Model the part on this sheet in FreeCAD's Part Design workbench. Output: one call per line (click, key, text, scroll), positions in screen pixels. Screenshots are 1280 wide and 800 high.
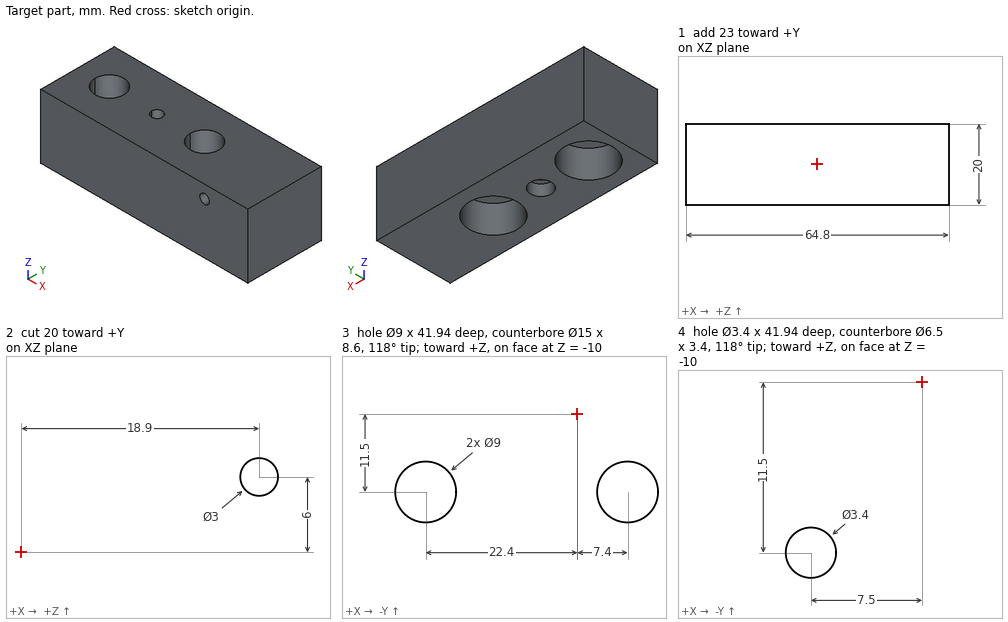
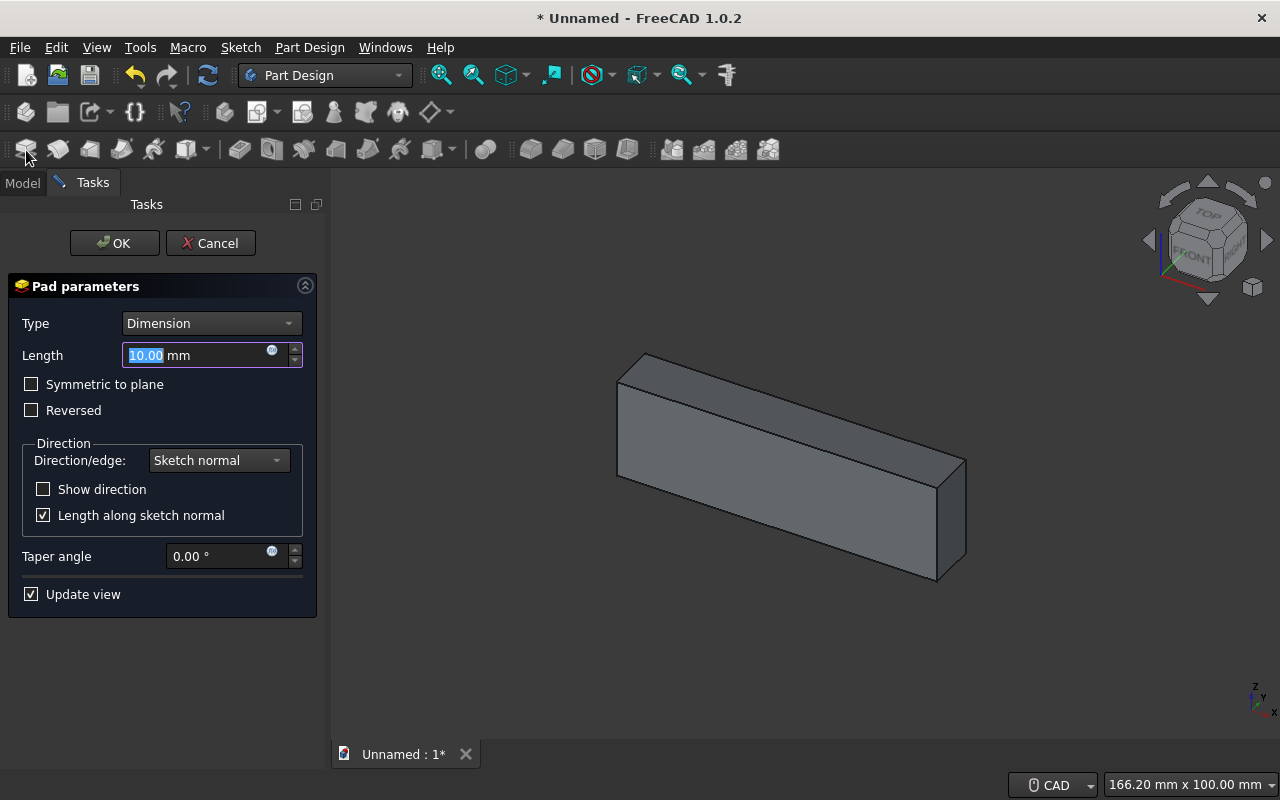
text(23)
key(Tab)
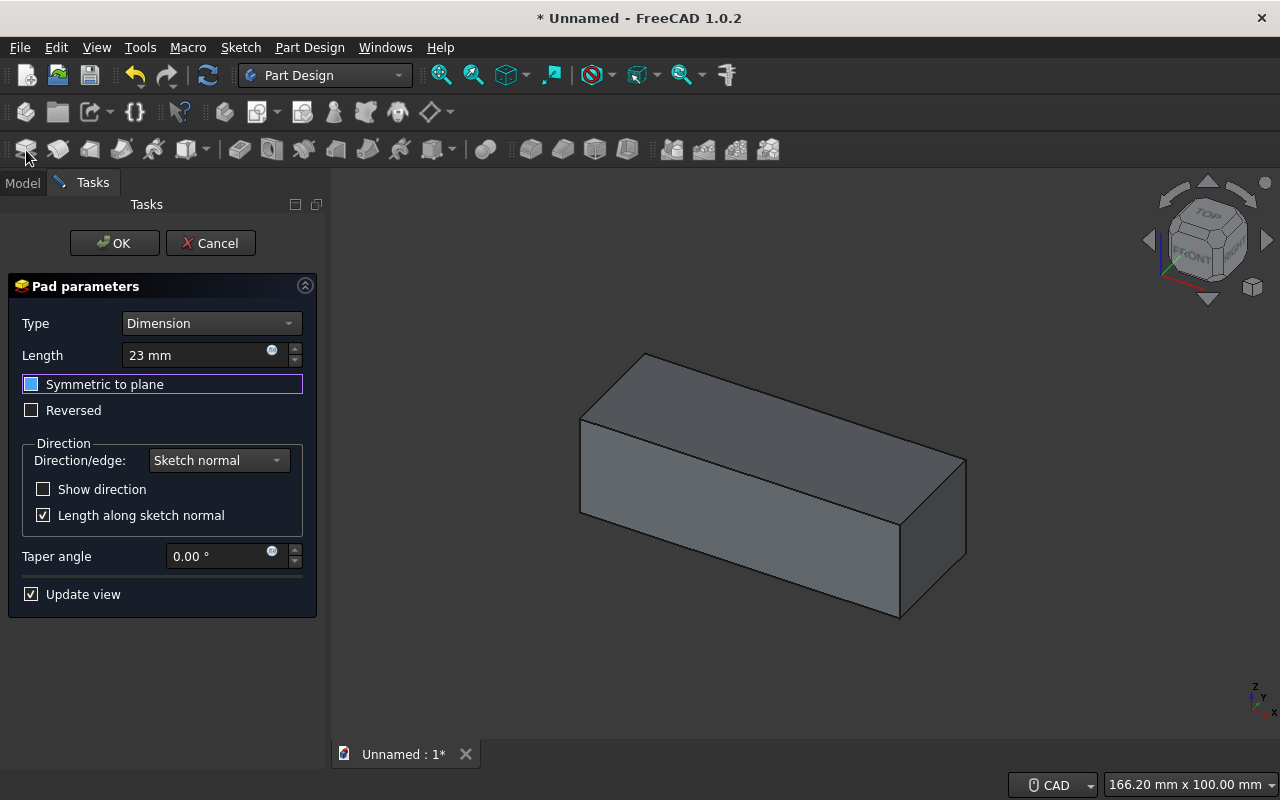
click(30, 410)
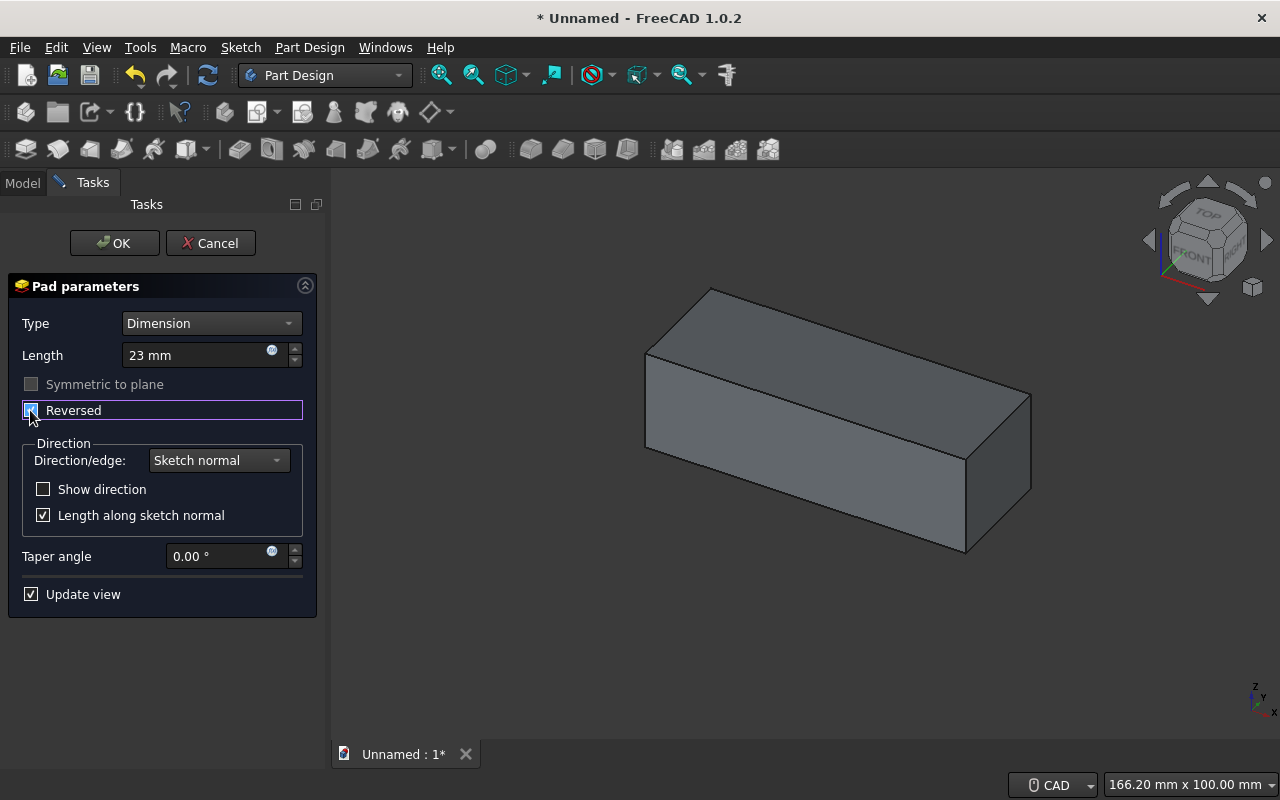
click(115, 243)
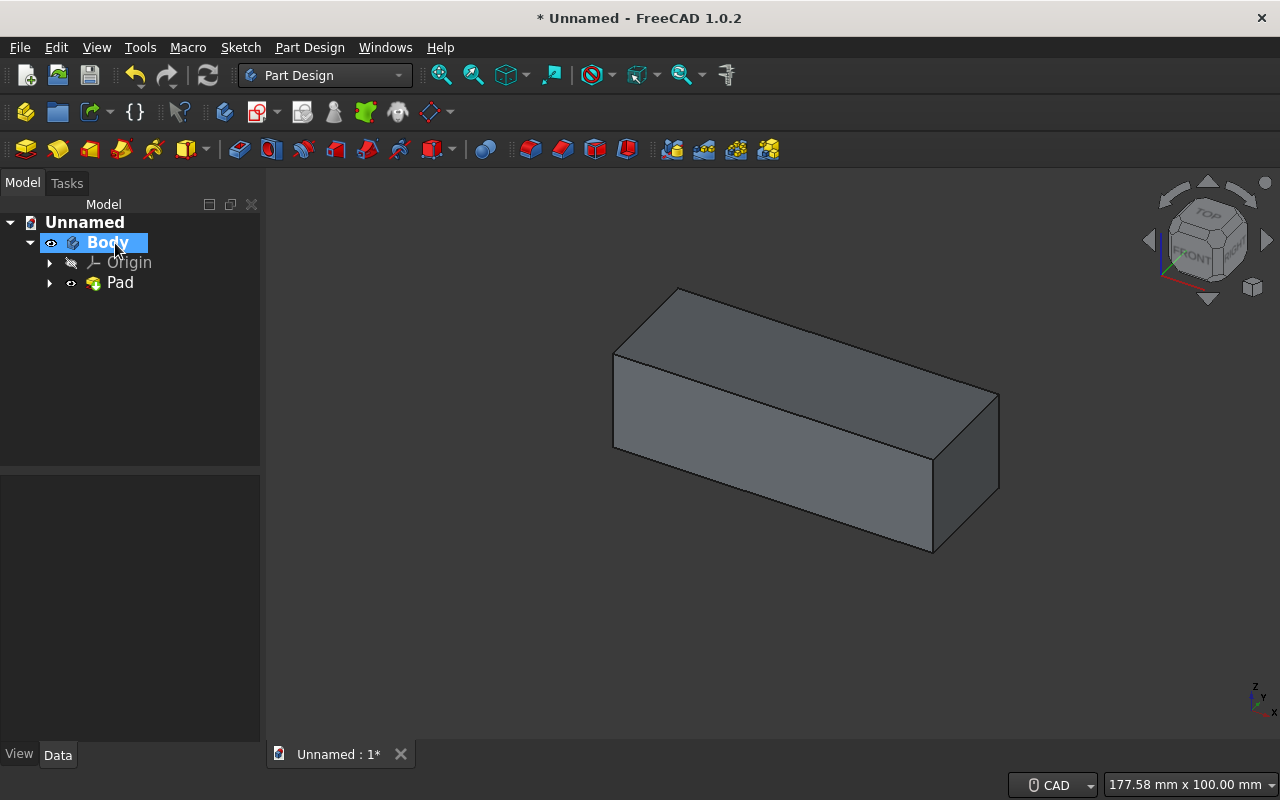
click(258, 112)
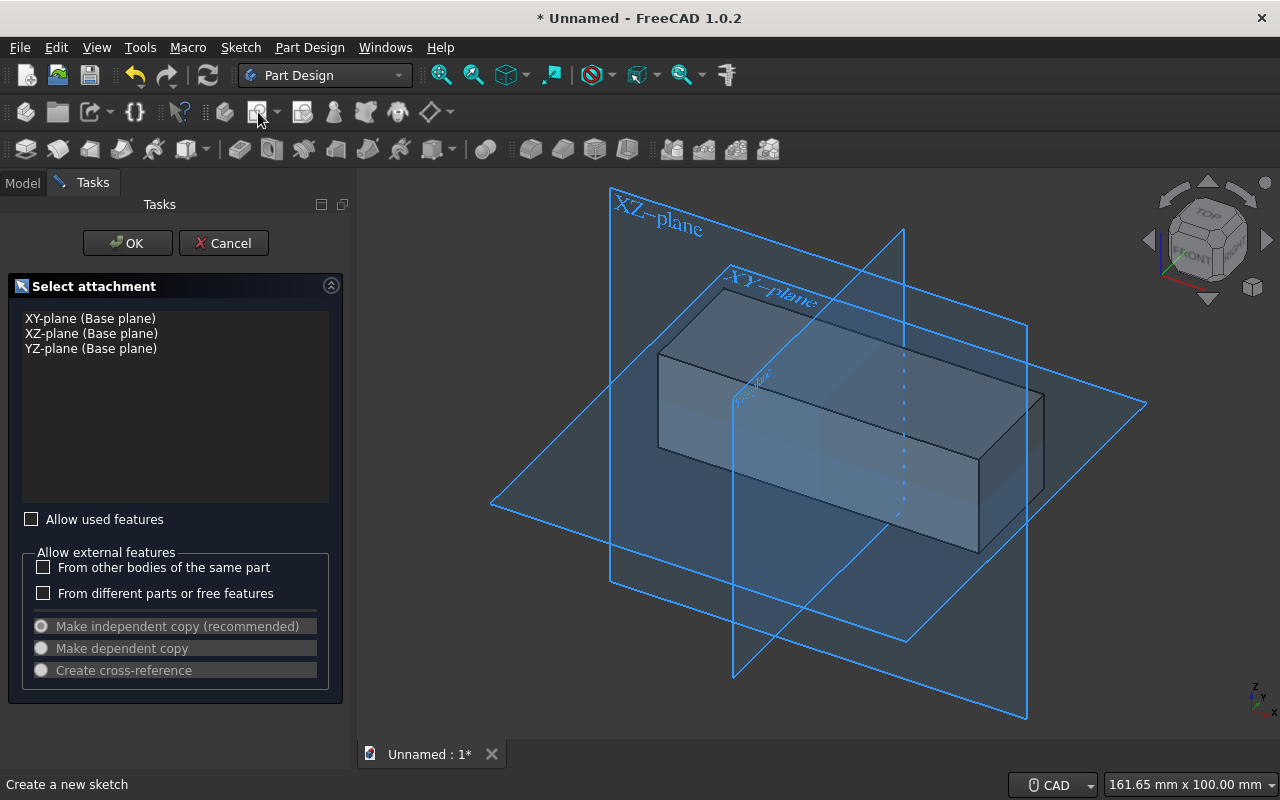
click(82, 334)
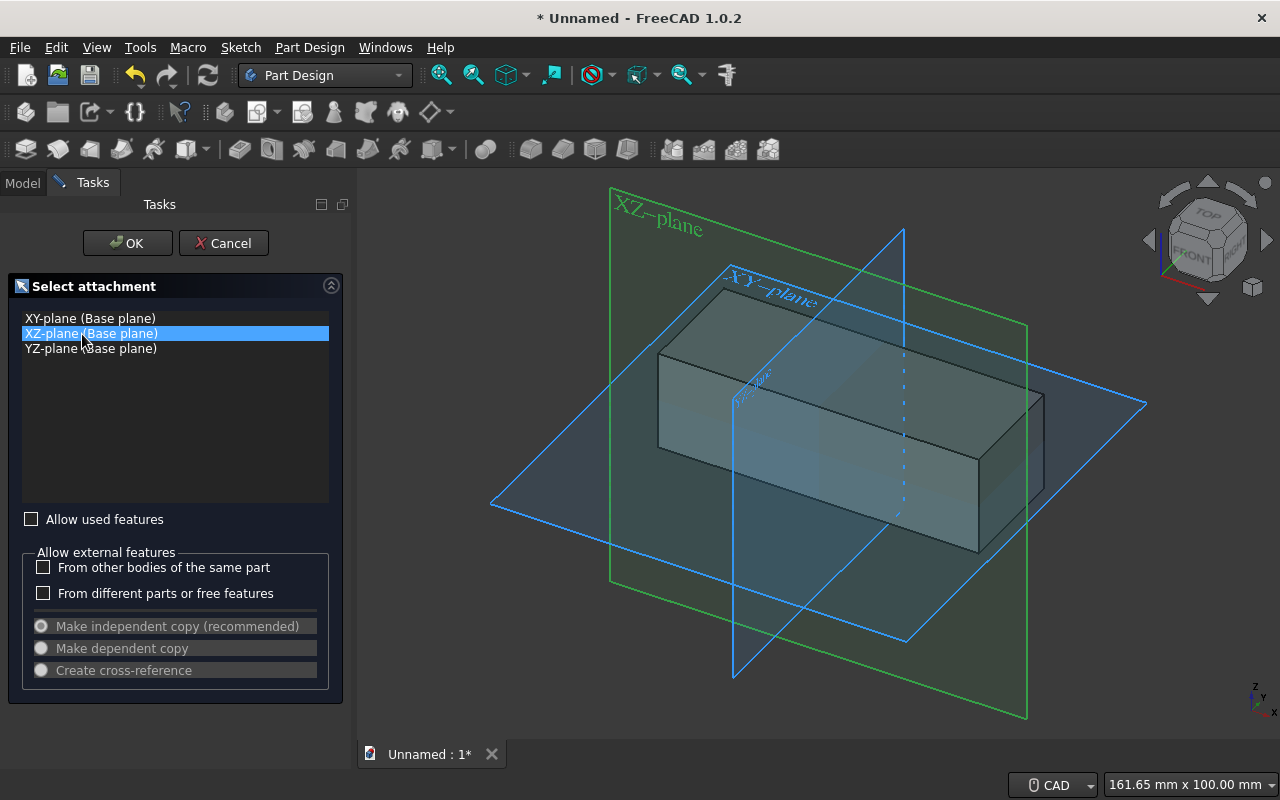
click(128, 243)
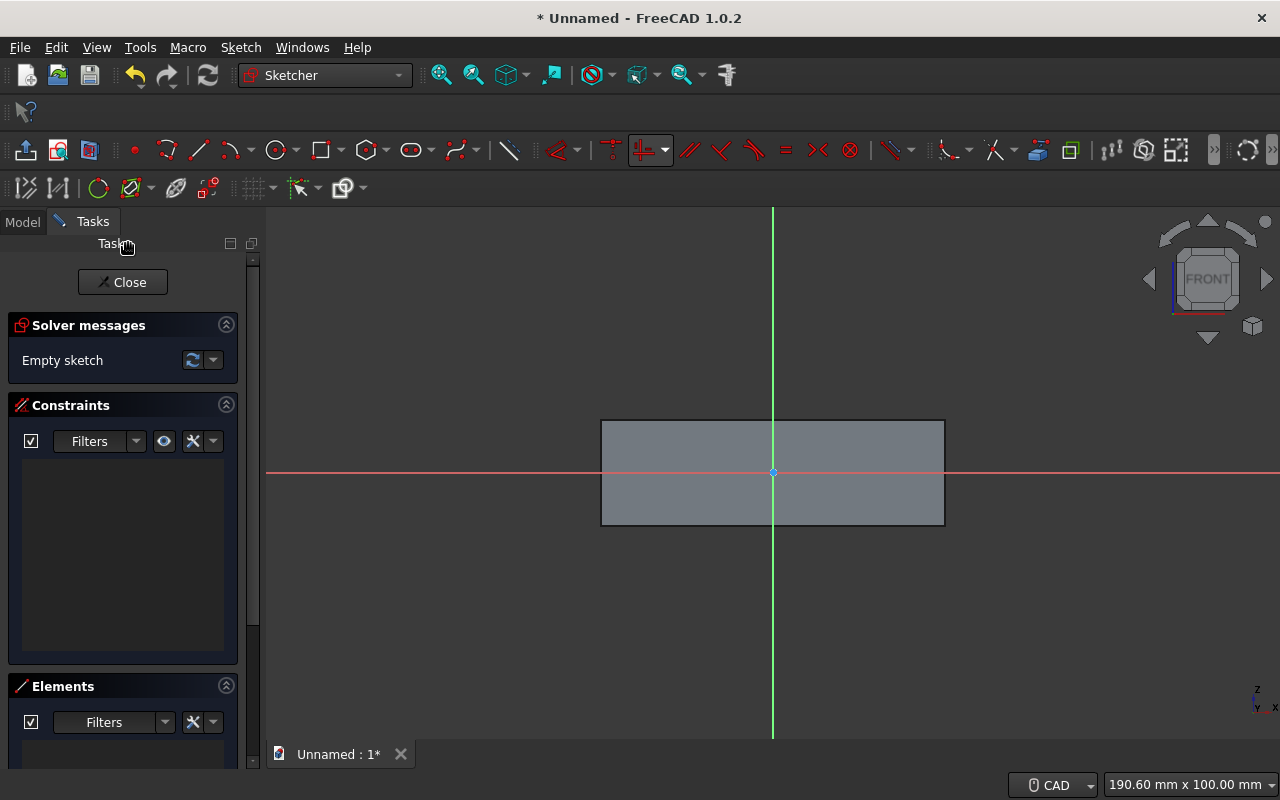
scroll(882, 439, up, 15)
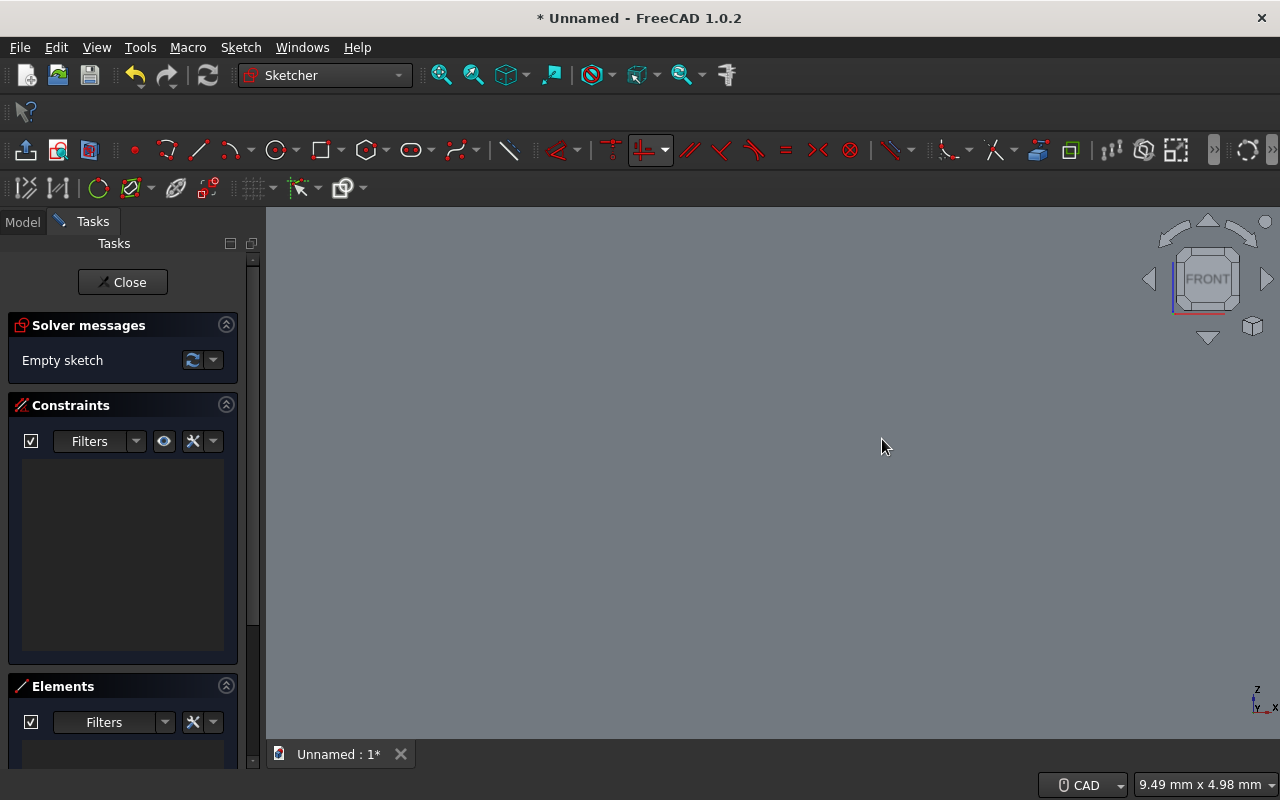
click(276, 150)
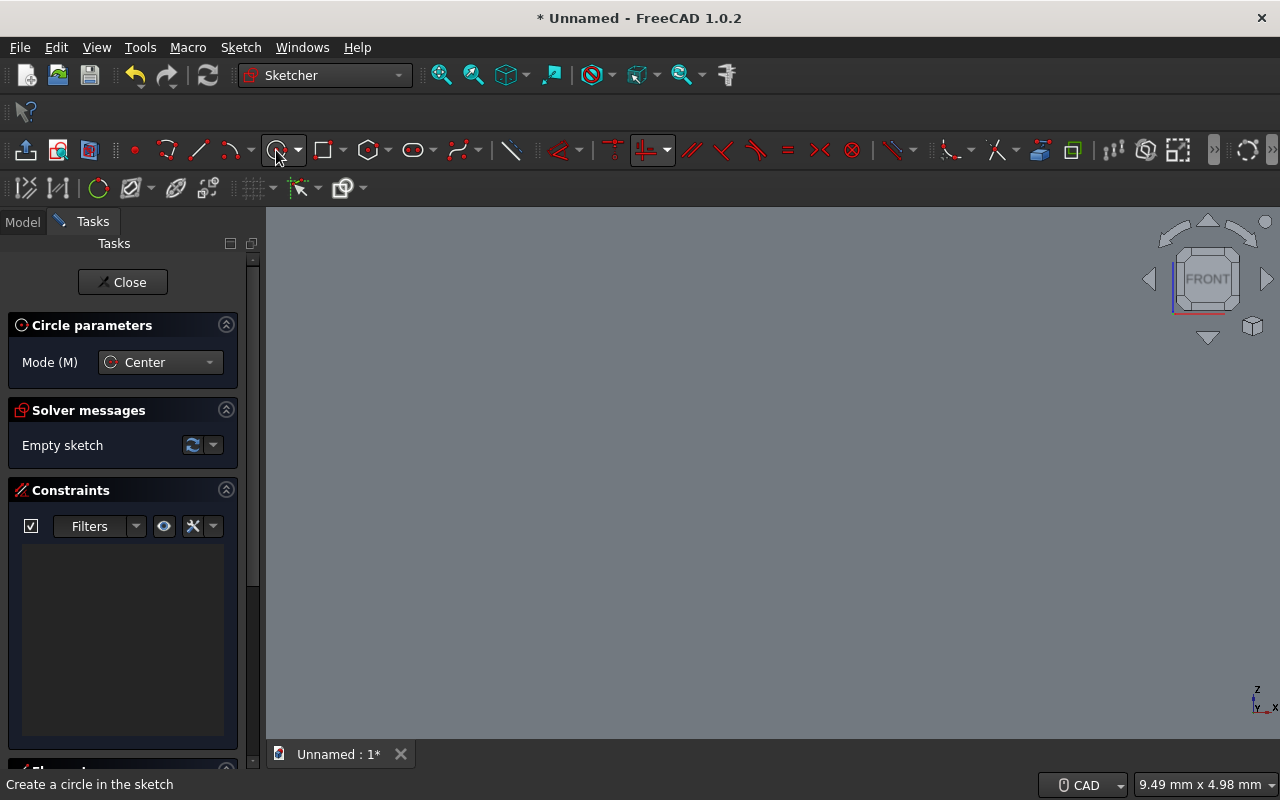
click(701, 472)
move(814, 359)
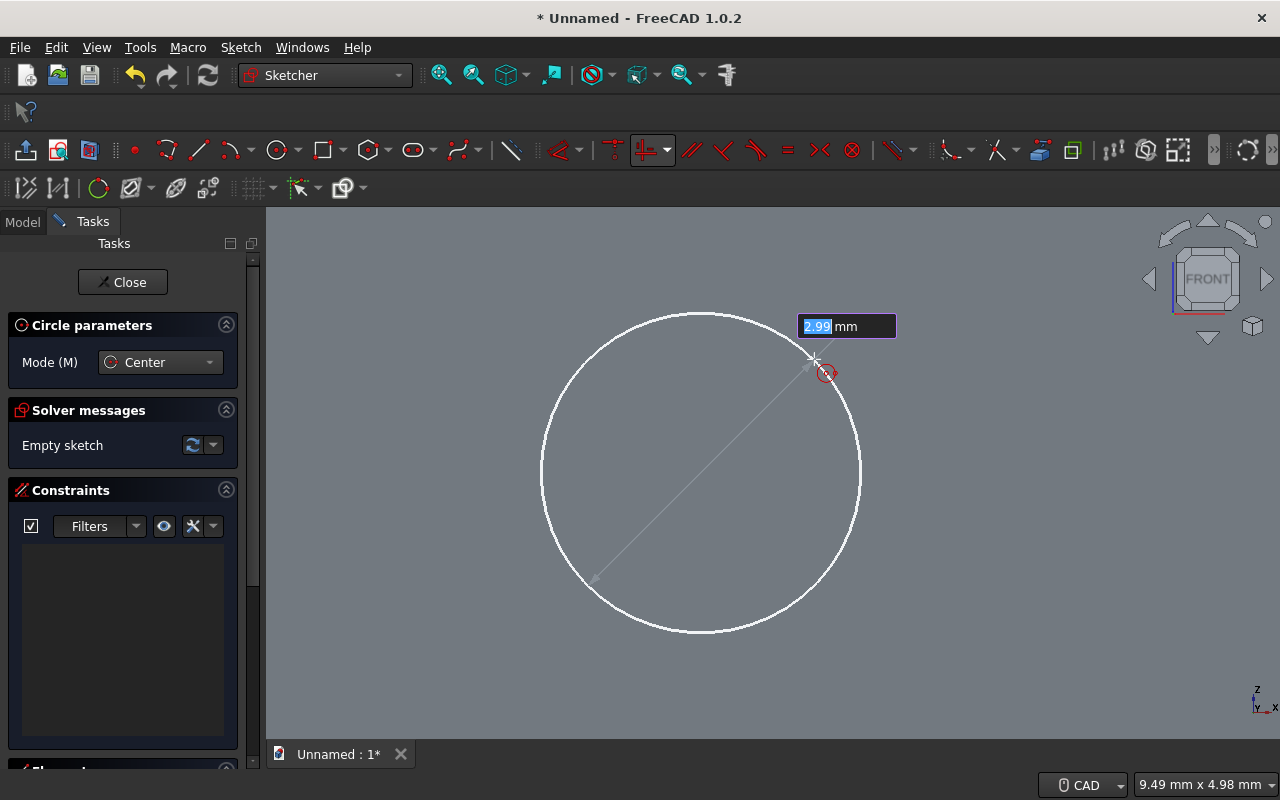
text(3)
key(Return)
key(Escape)